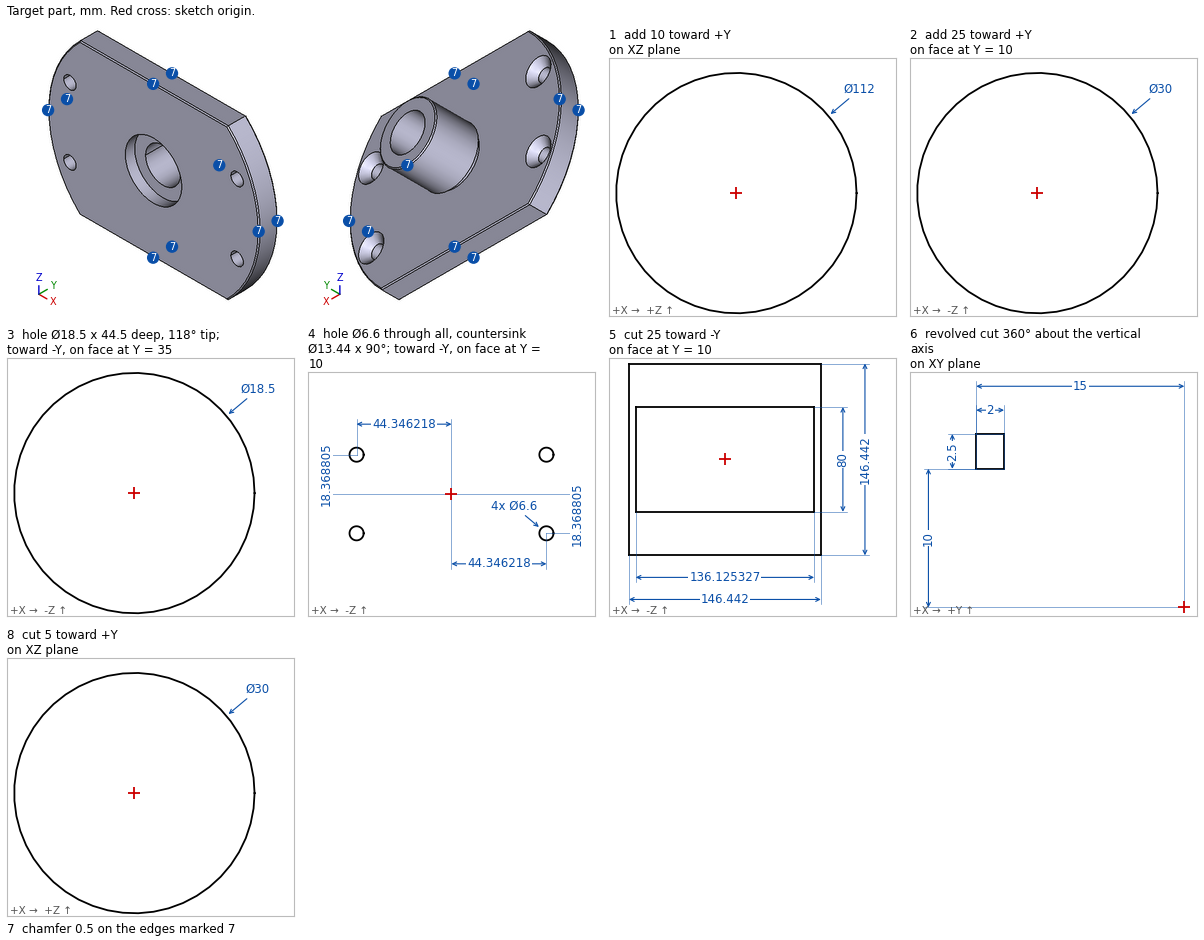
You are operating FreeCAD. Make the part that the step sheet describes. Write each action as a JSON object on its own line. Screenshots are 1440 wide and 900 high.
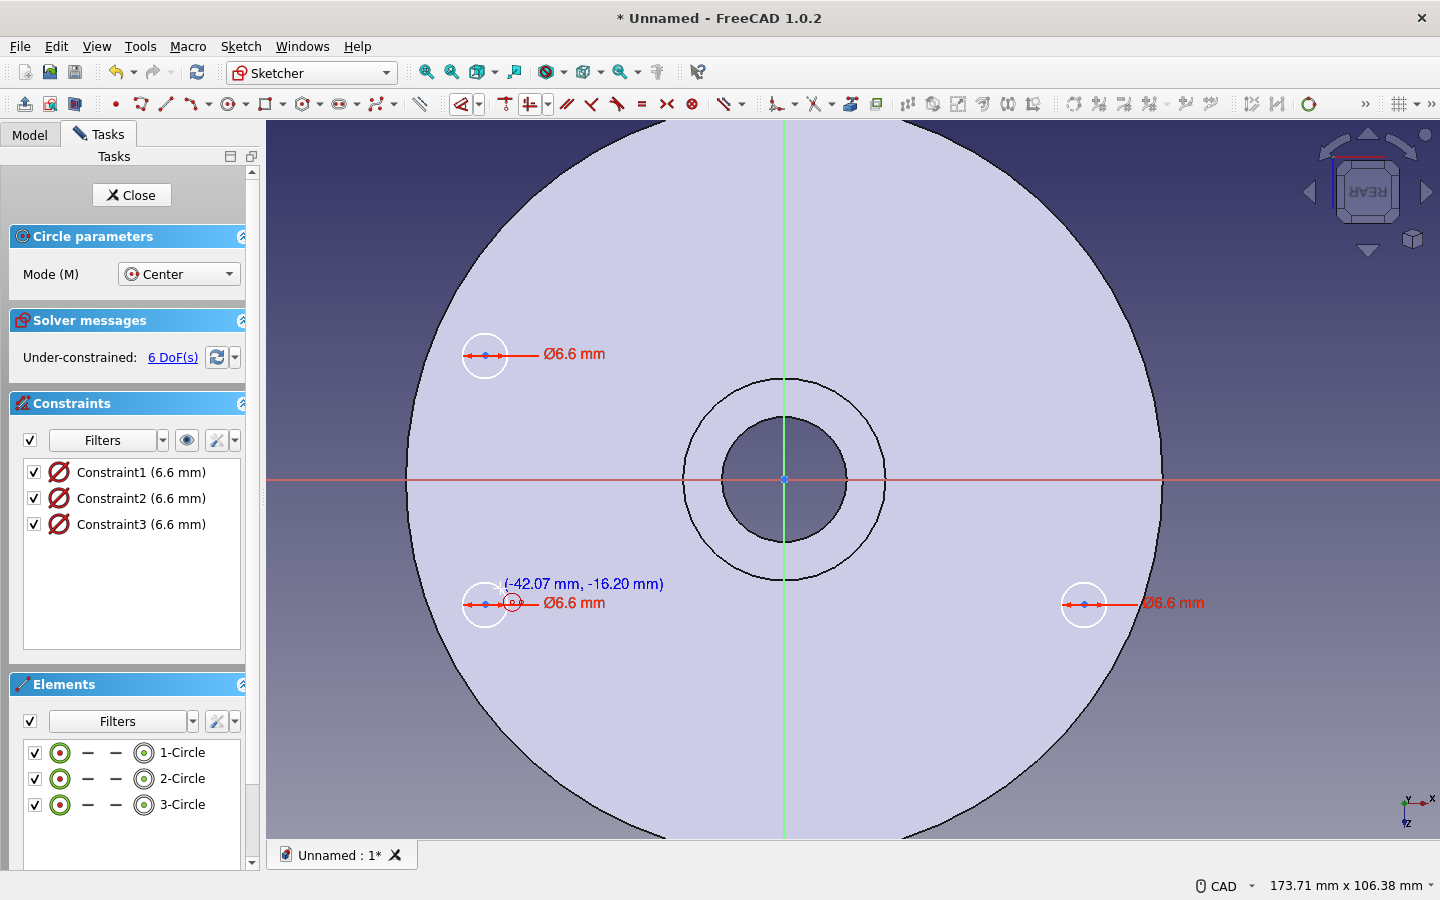
{"action": "left_click", "coordinate": [1084, 355]}
{"action": "mouse_move", "coordinate": [1100, 340]}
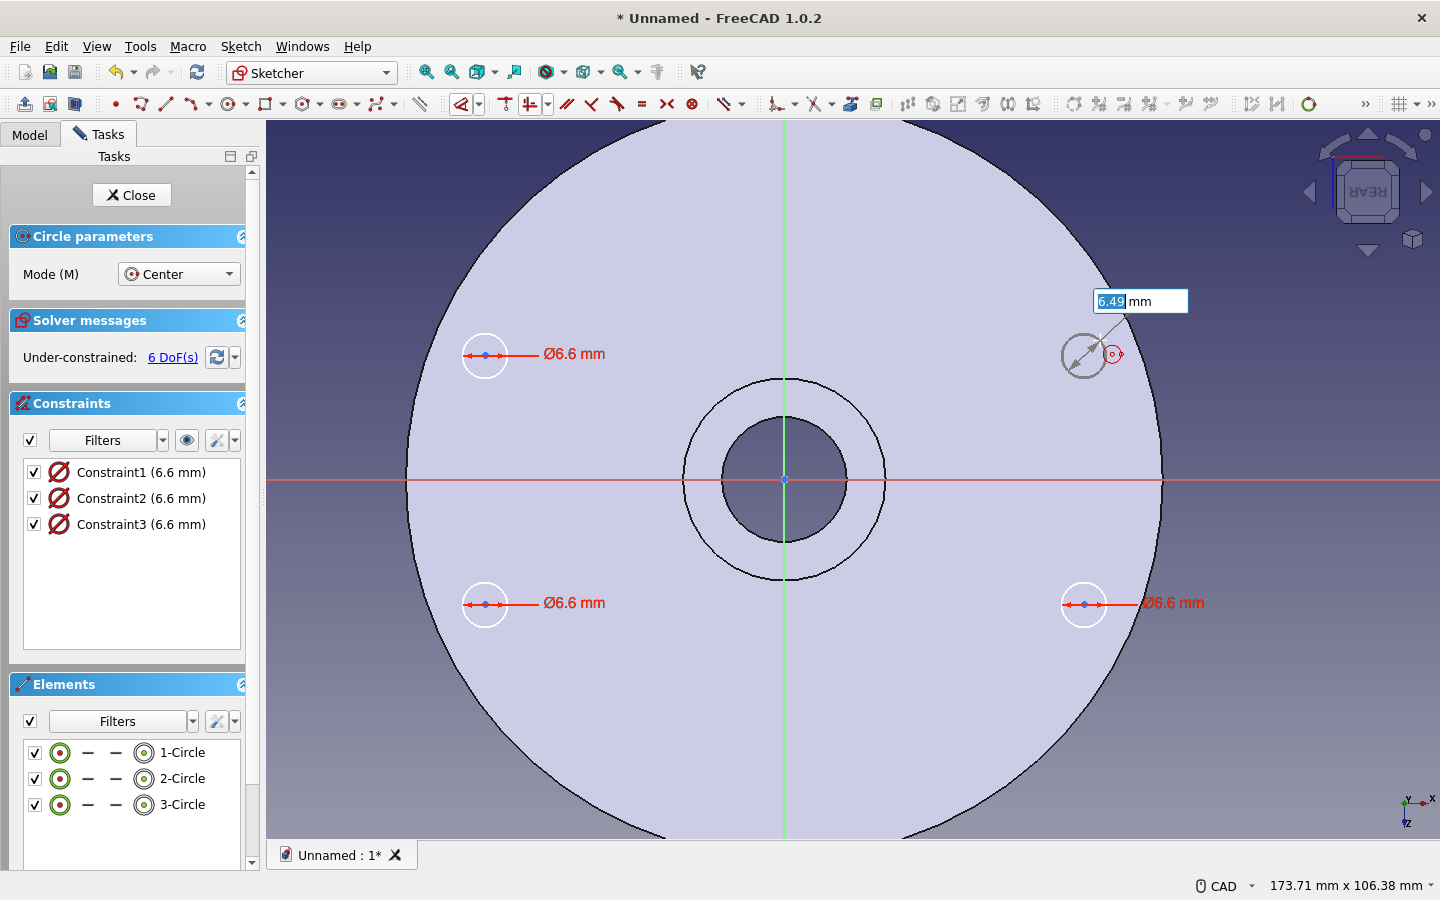
{"action": "type", "text": "6.6"}
{"action": "key", "text": "Return"}
{"action": "key", "text": "Escape"}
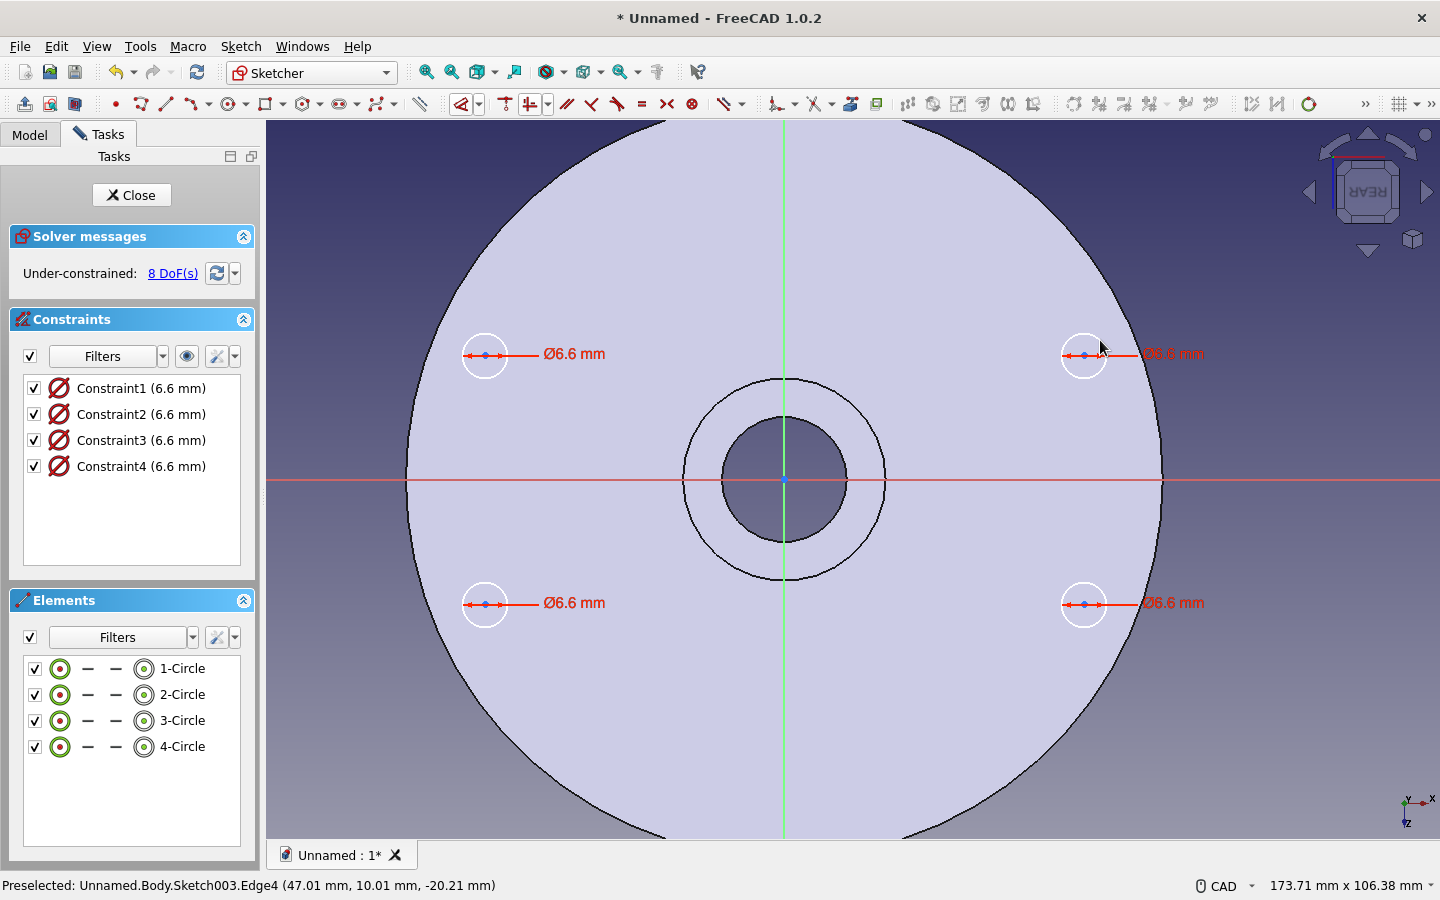
{"action": "left_click", "coordinate": [485, 356]}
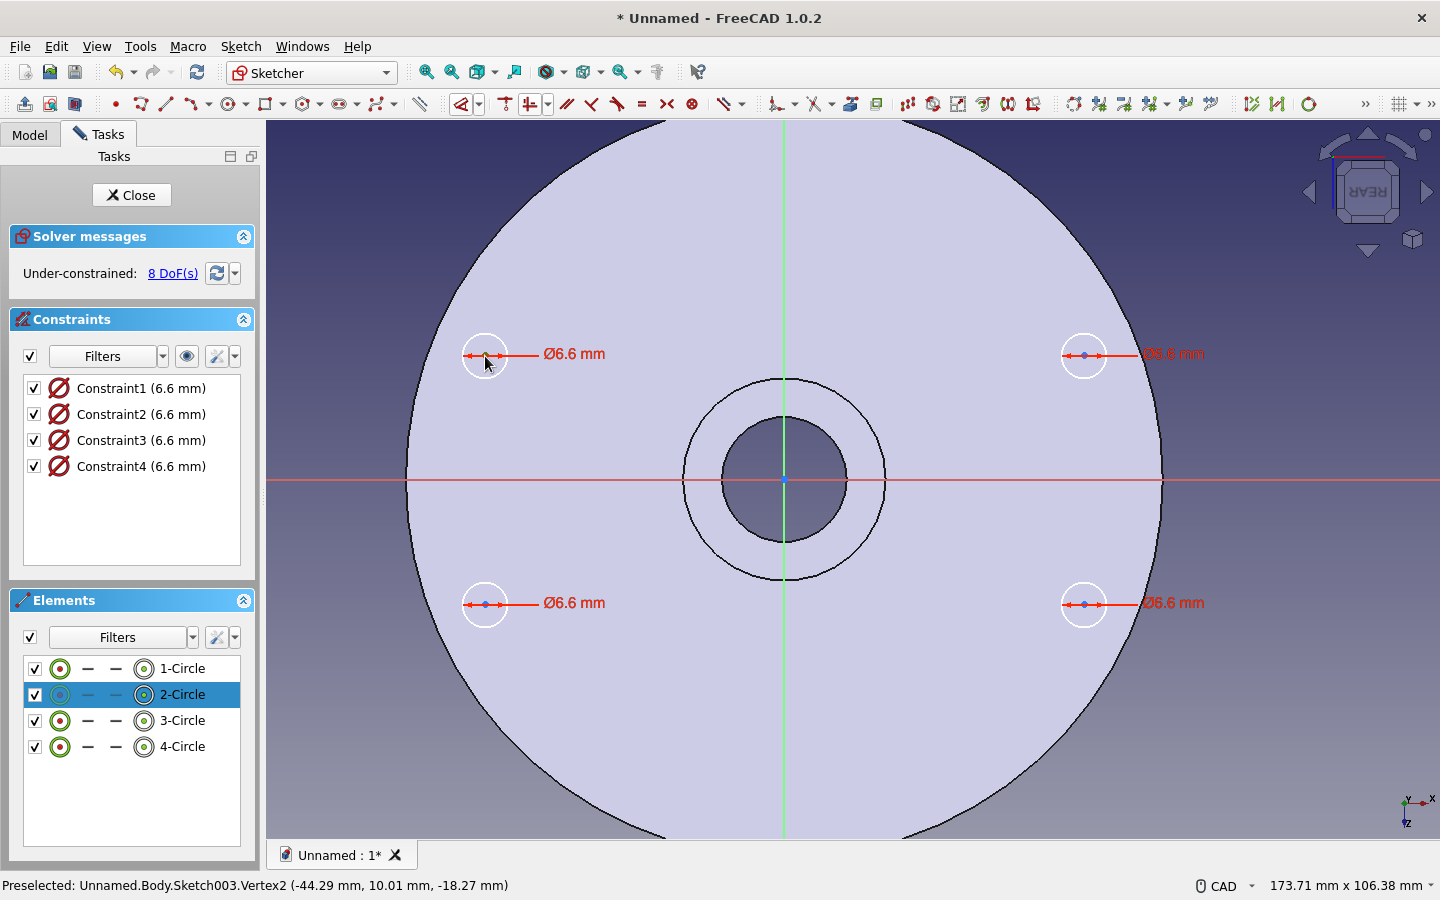
{"action": "left_click", "coordinate": [485, 605]}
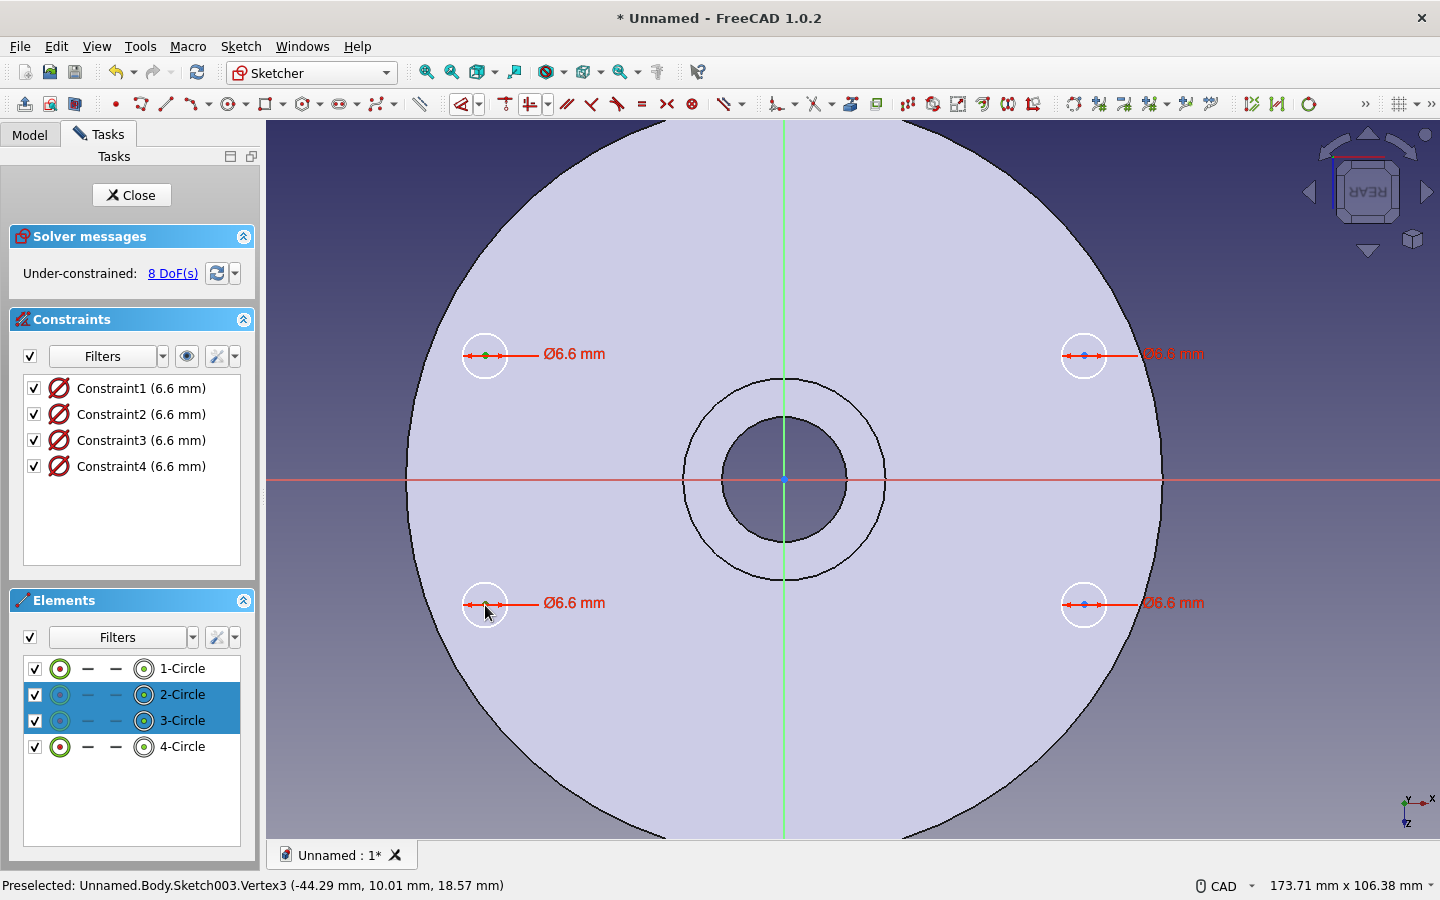
{"action": "key", "text": "v"}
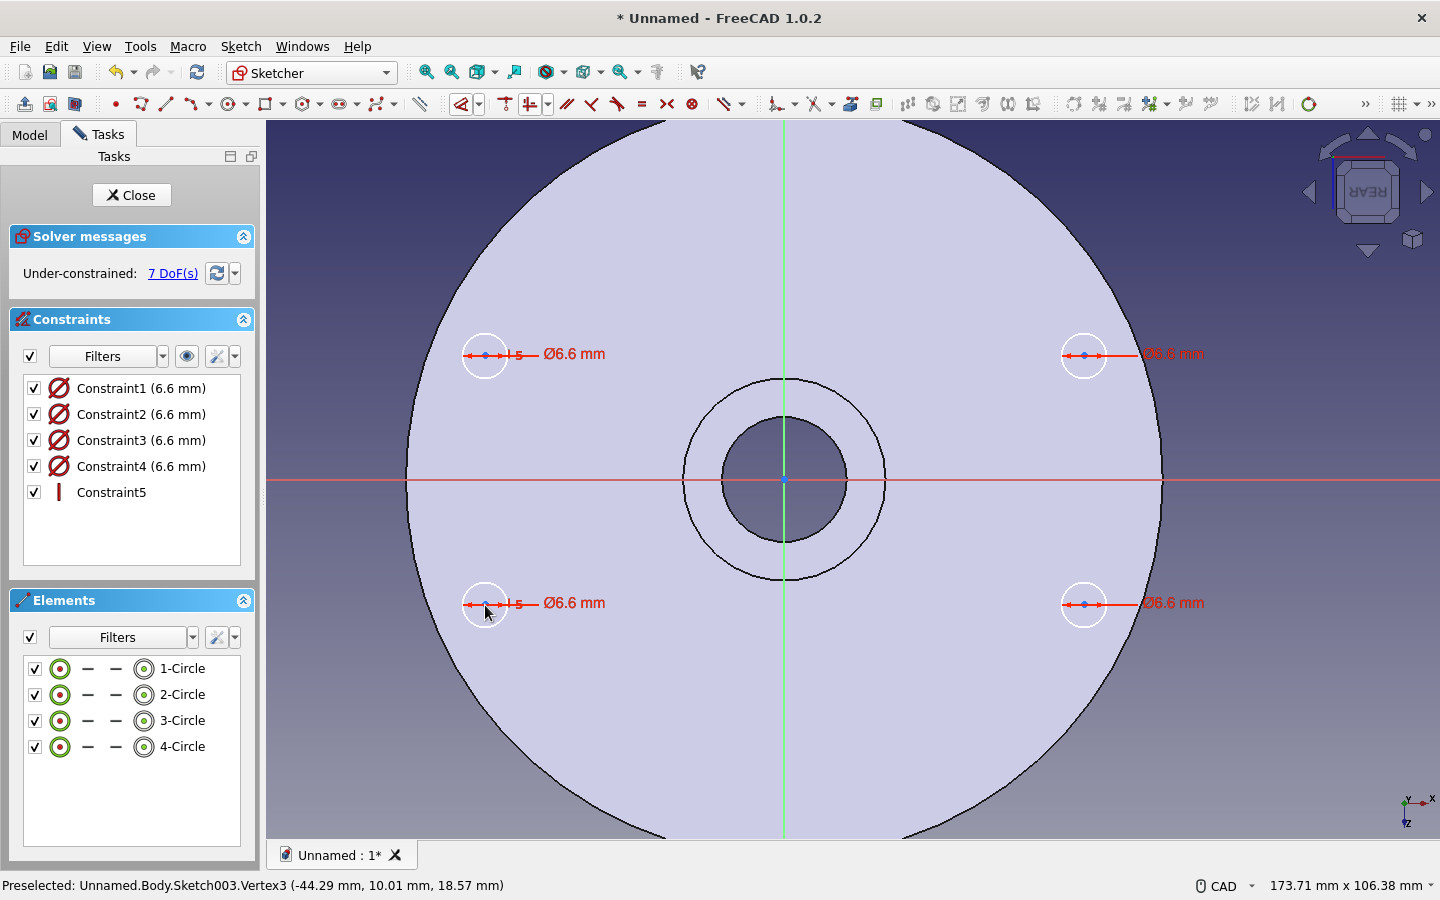
{"action": "left_click", "coordinate": [1084, 605]}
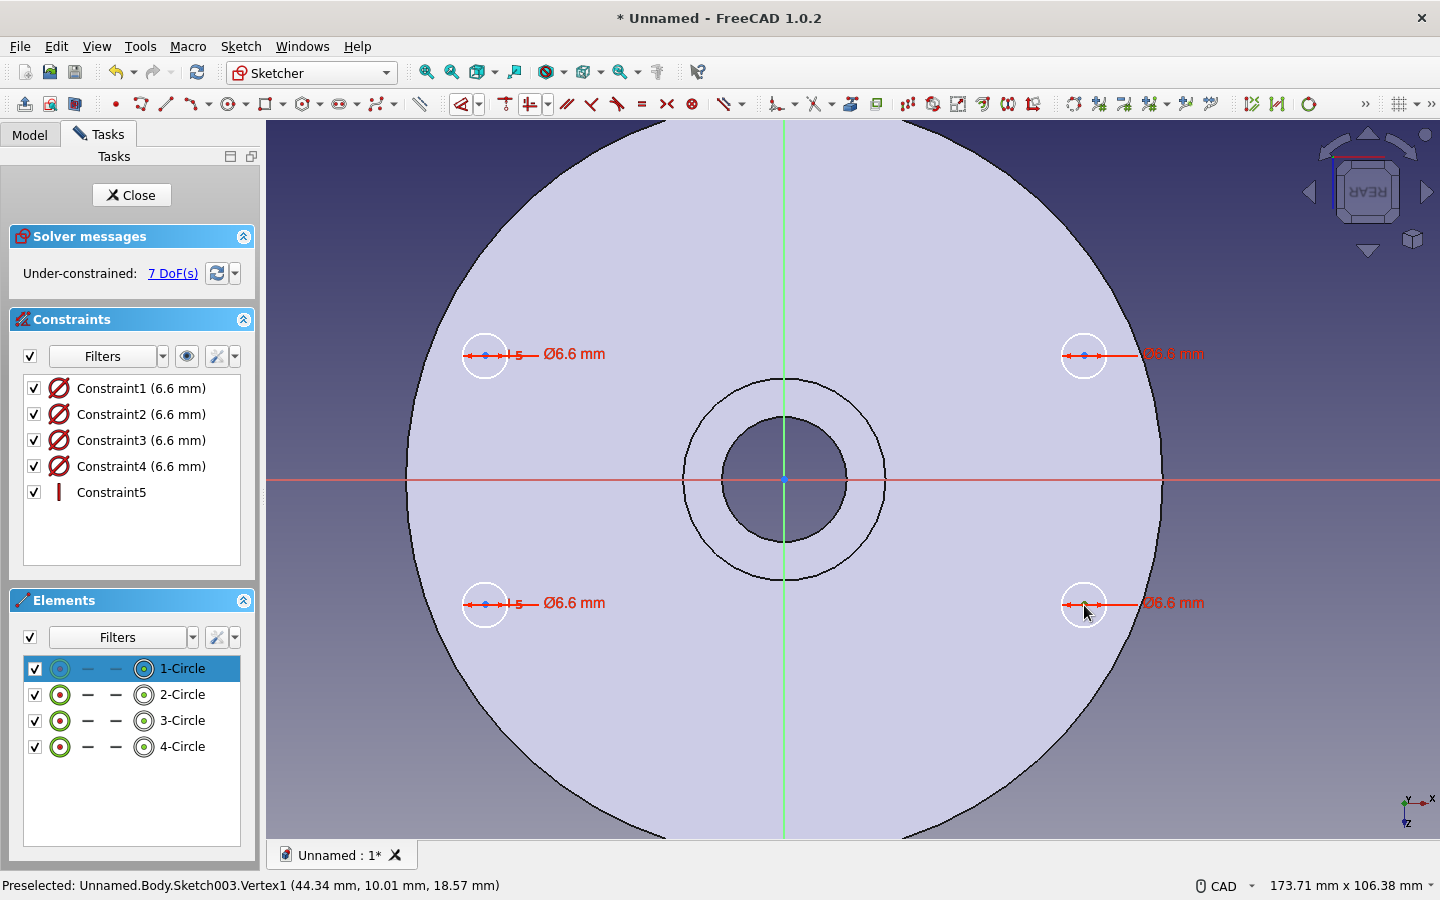
{"action": "left_click", "coordinate": [485, 605]}